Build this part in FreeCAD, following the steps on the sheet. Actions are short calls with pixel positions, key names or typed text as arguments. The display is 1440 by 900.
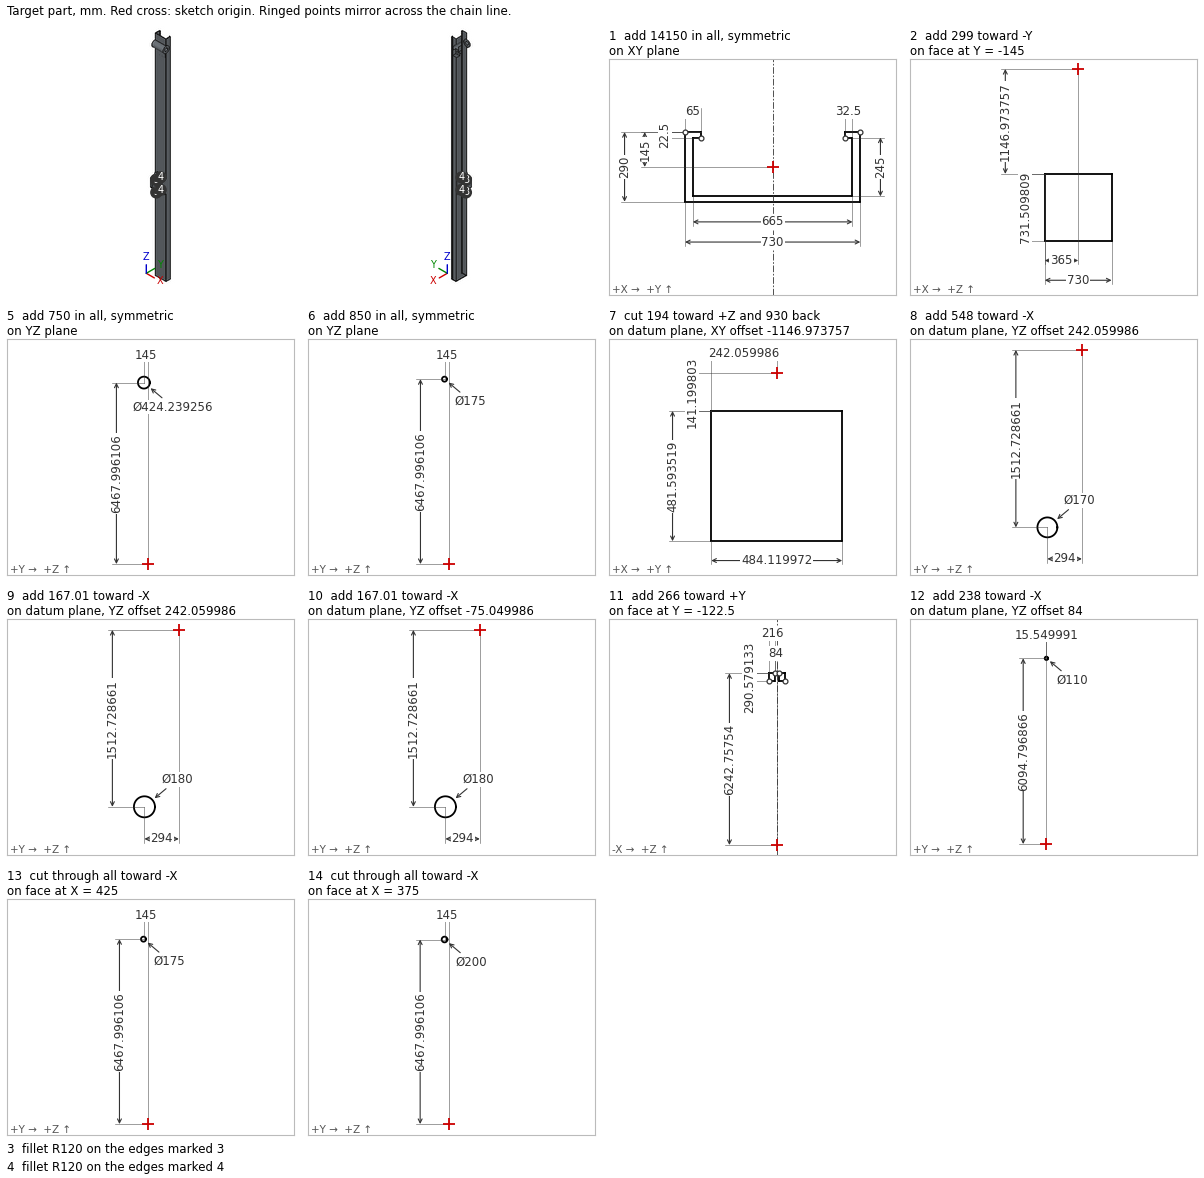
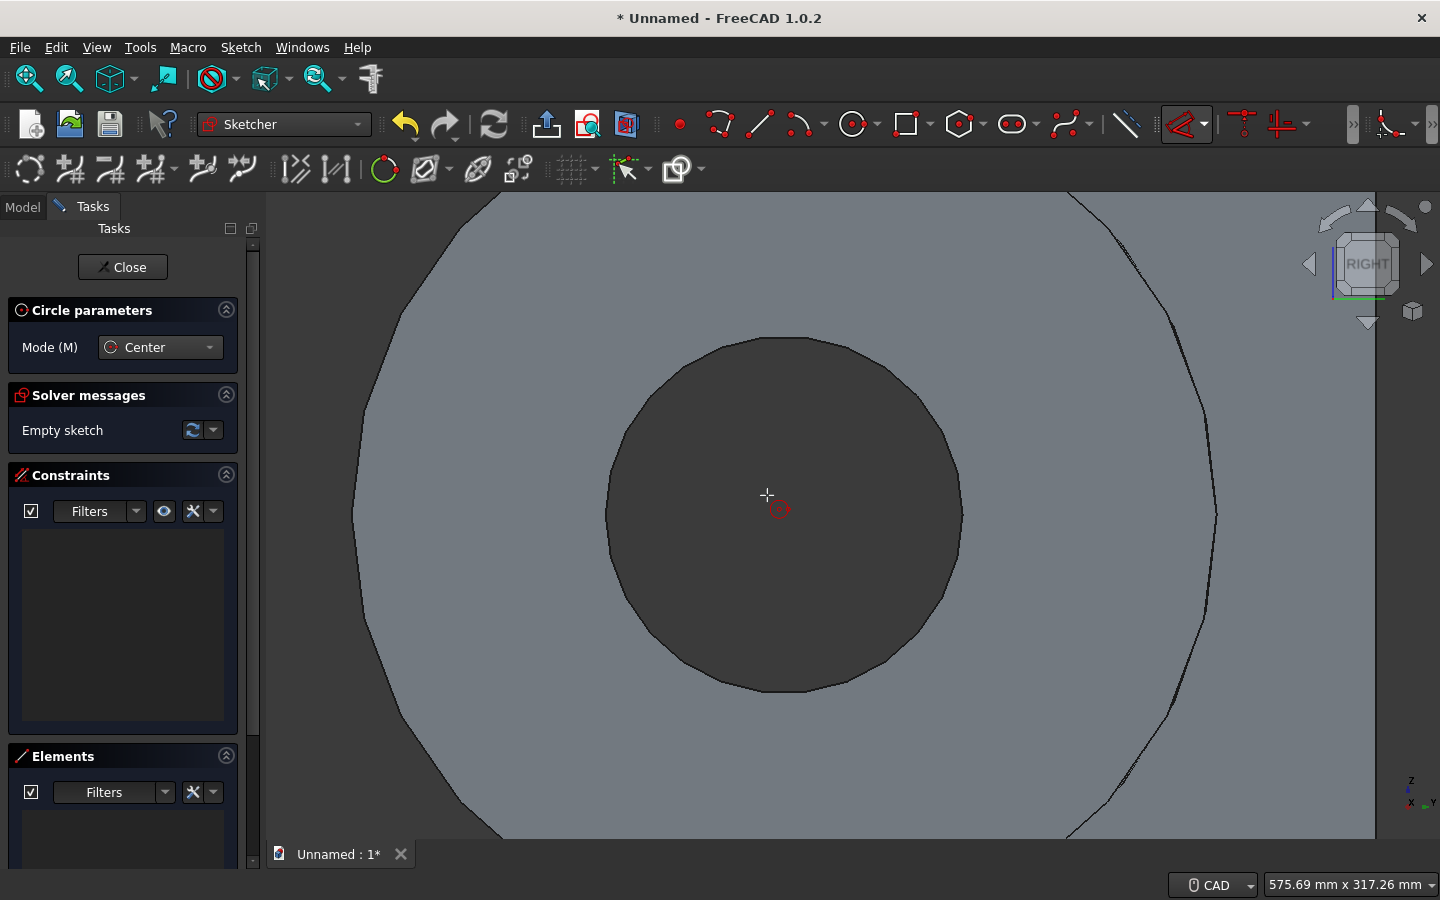
click(784, 515)
click(928, 371)
key(Escape)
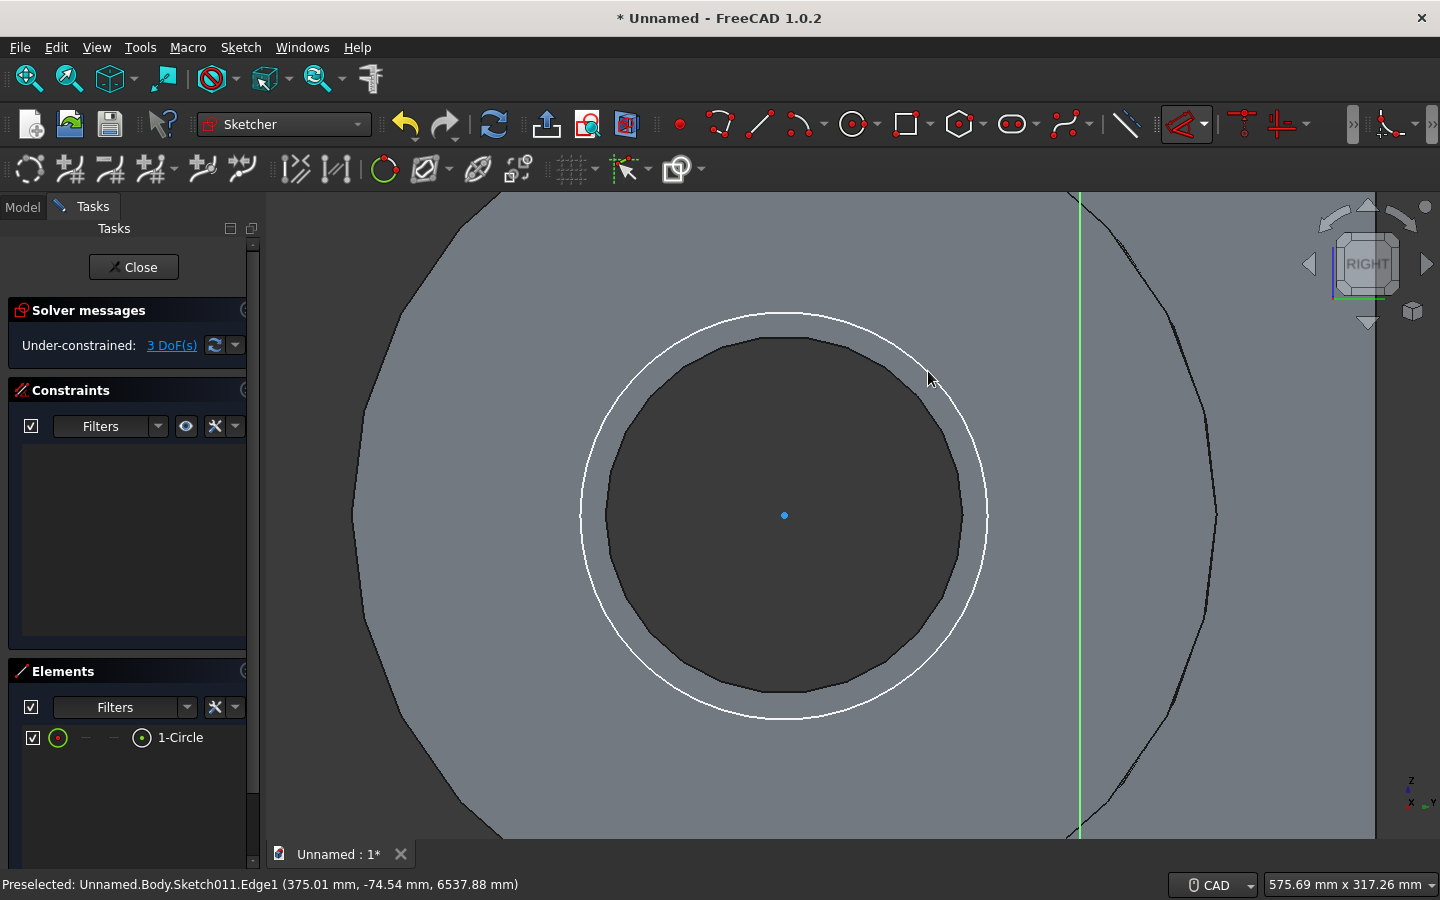
click(928, 372)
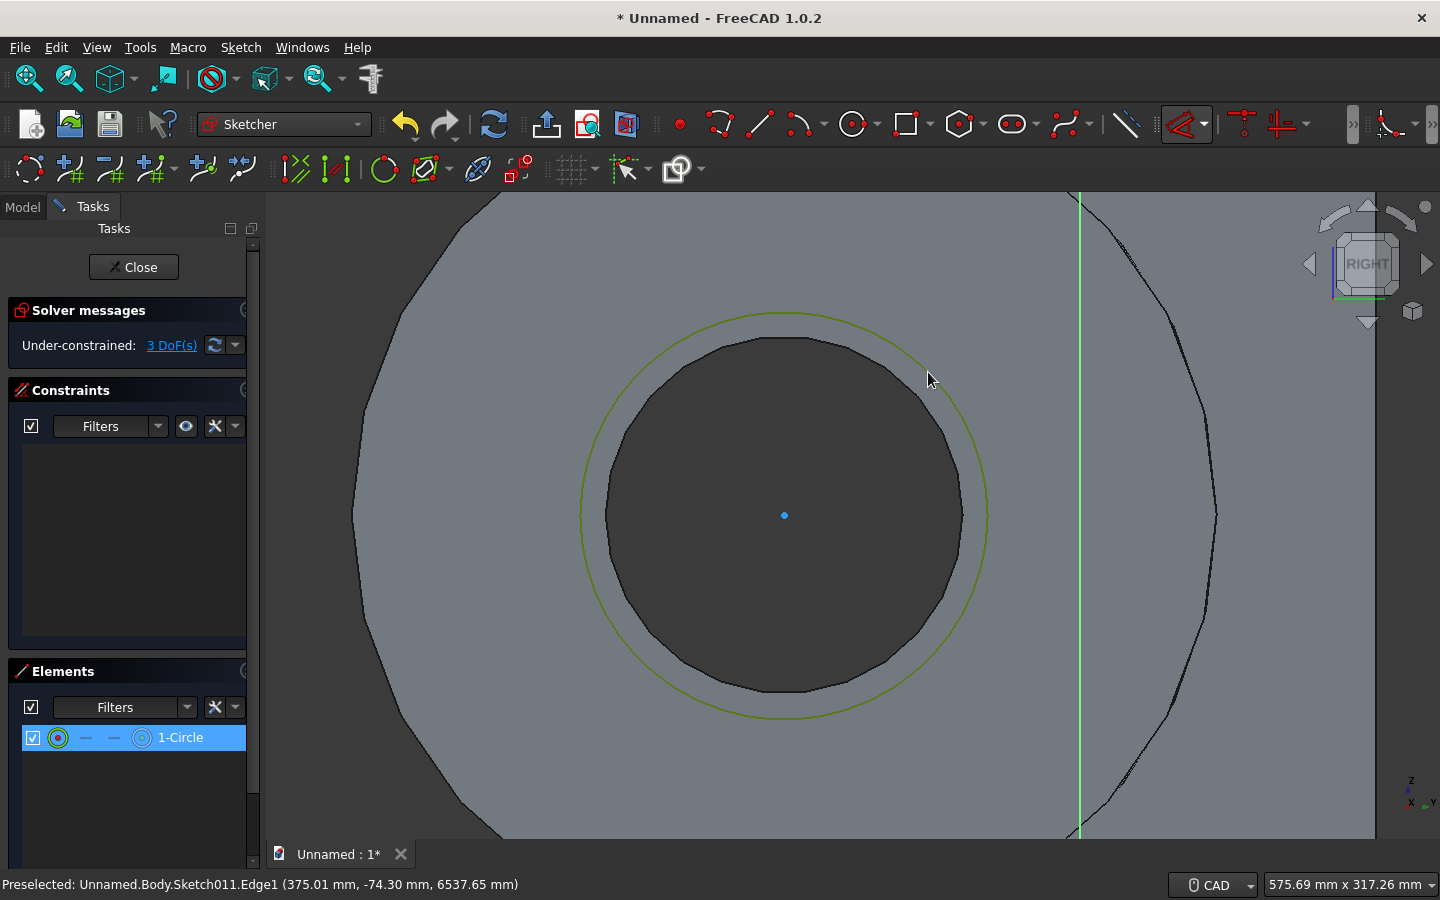
key(k)
key(o)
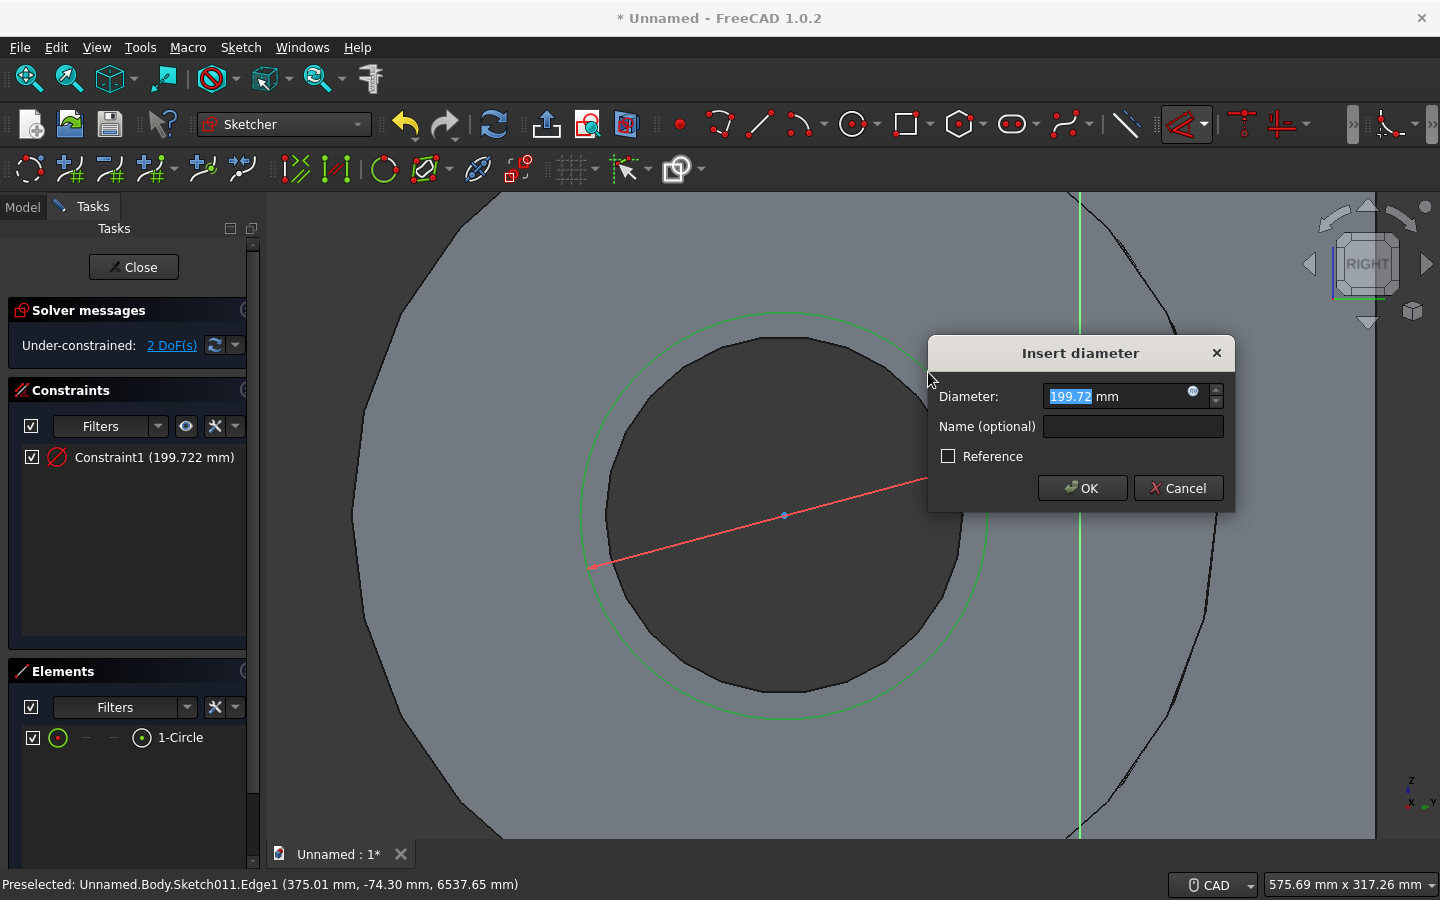
text(200)
key(Return)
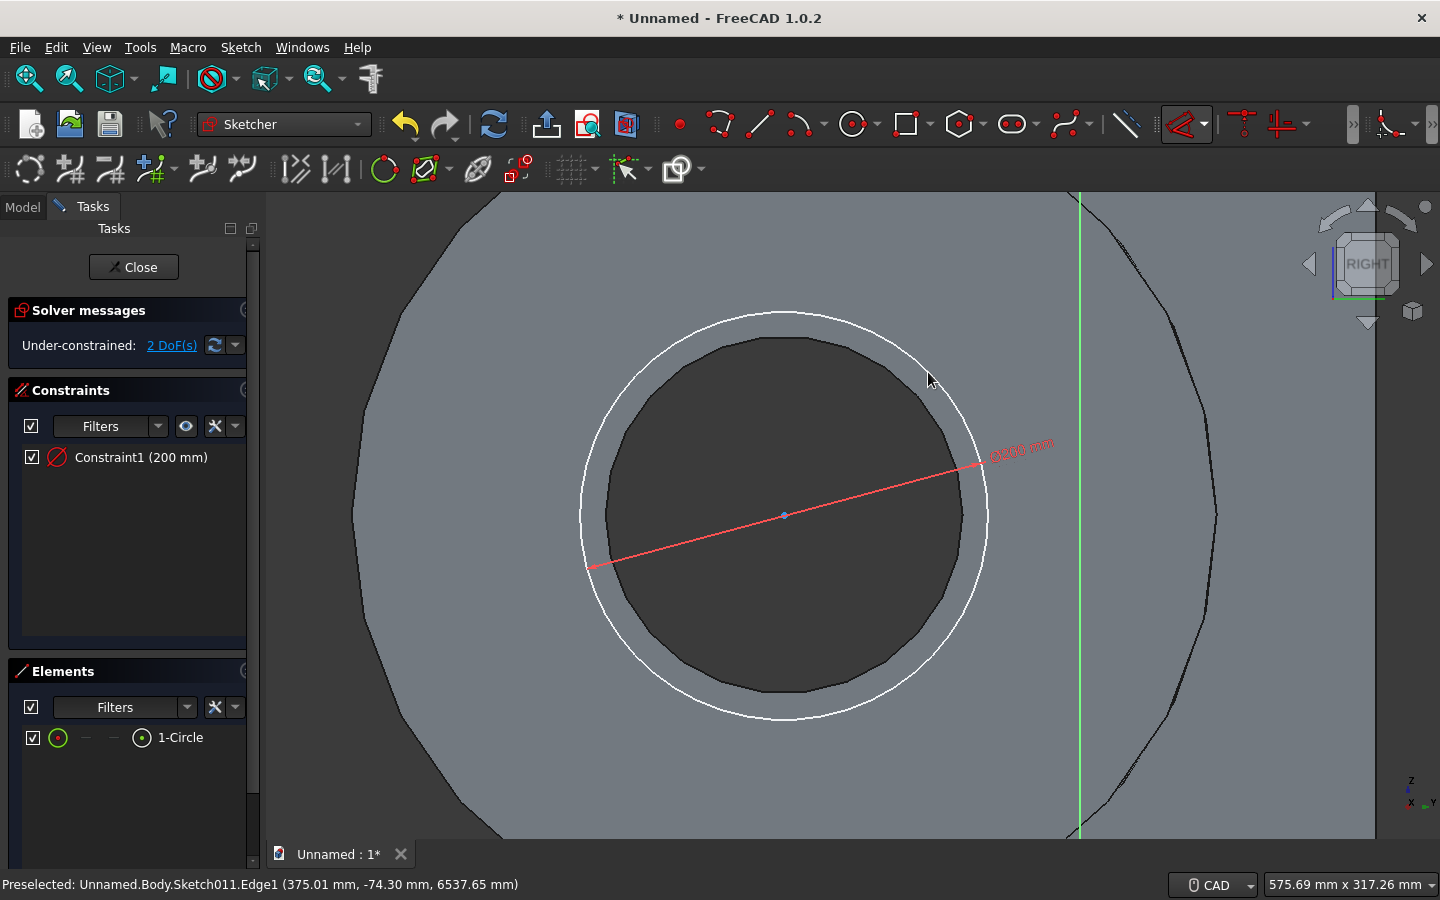
click(784, 516)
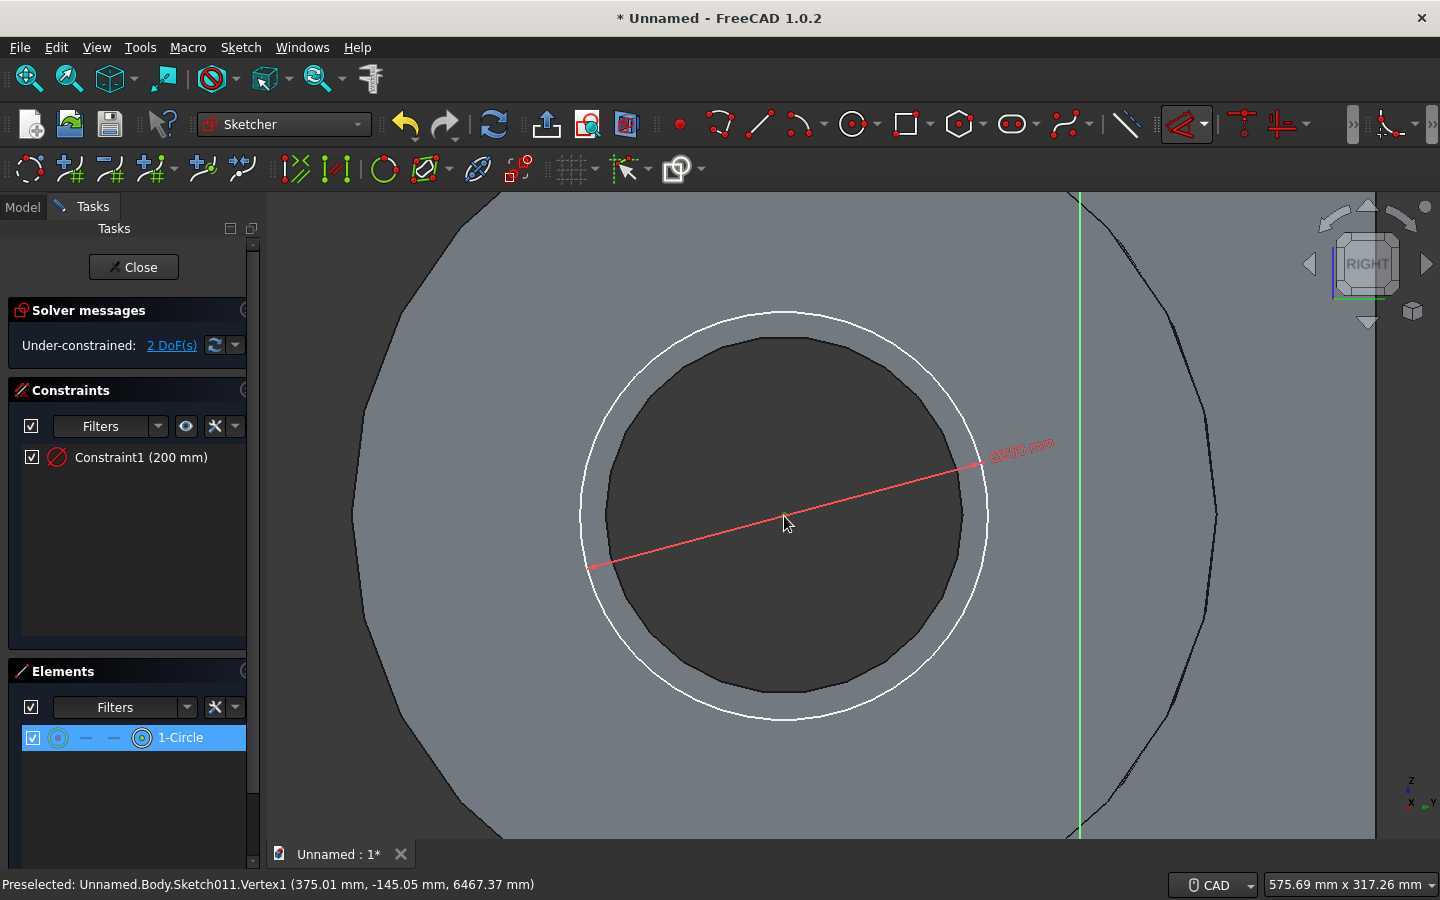
key(l)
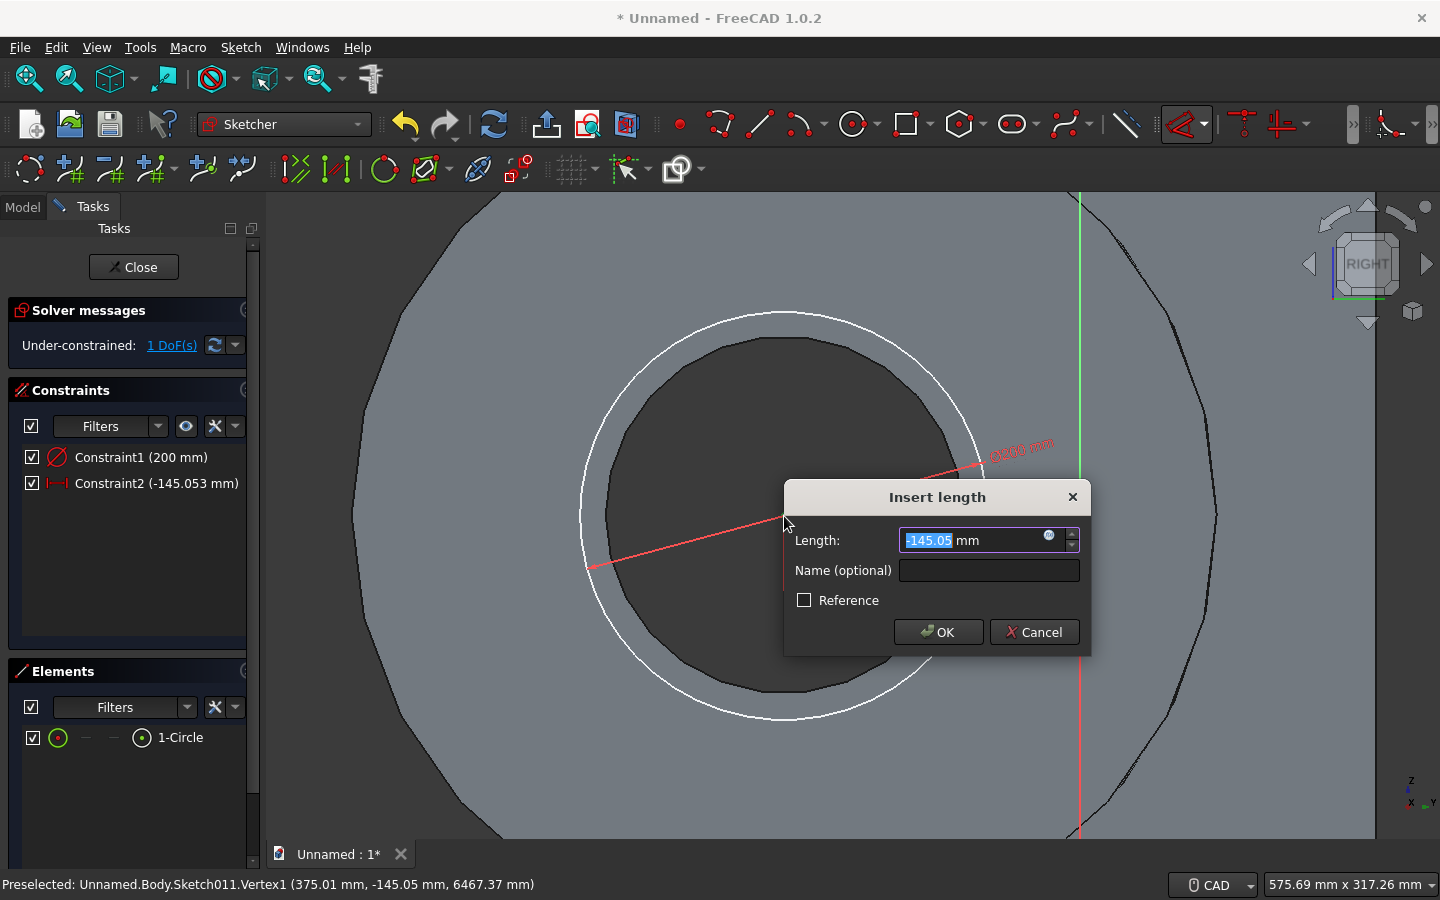
text(-145)
key(Return)